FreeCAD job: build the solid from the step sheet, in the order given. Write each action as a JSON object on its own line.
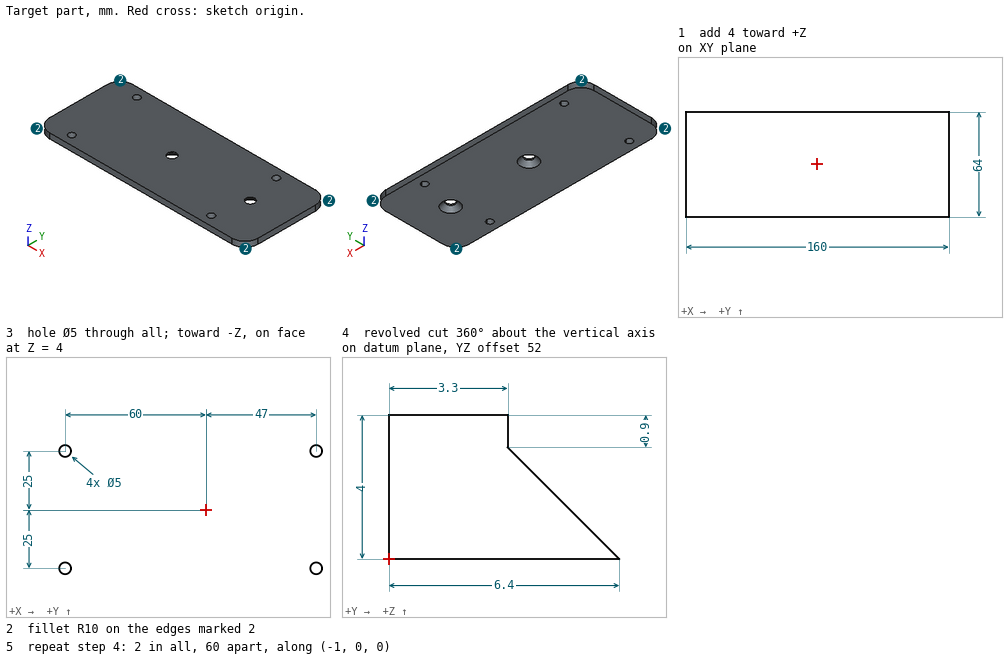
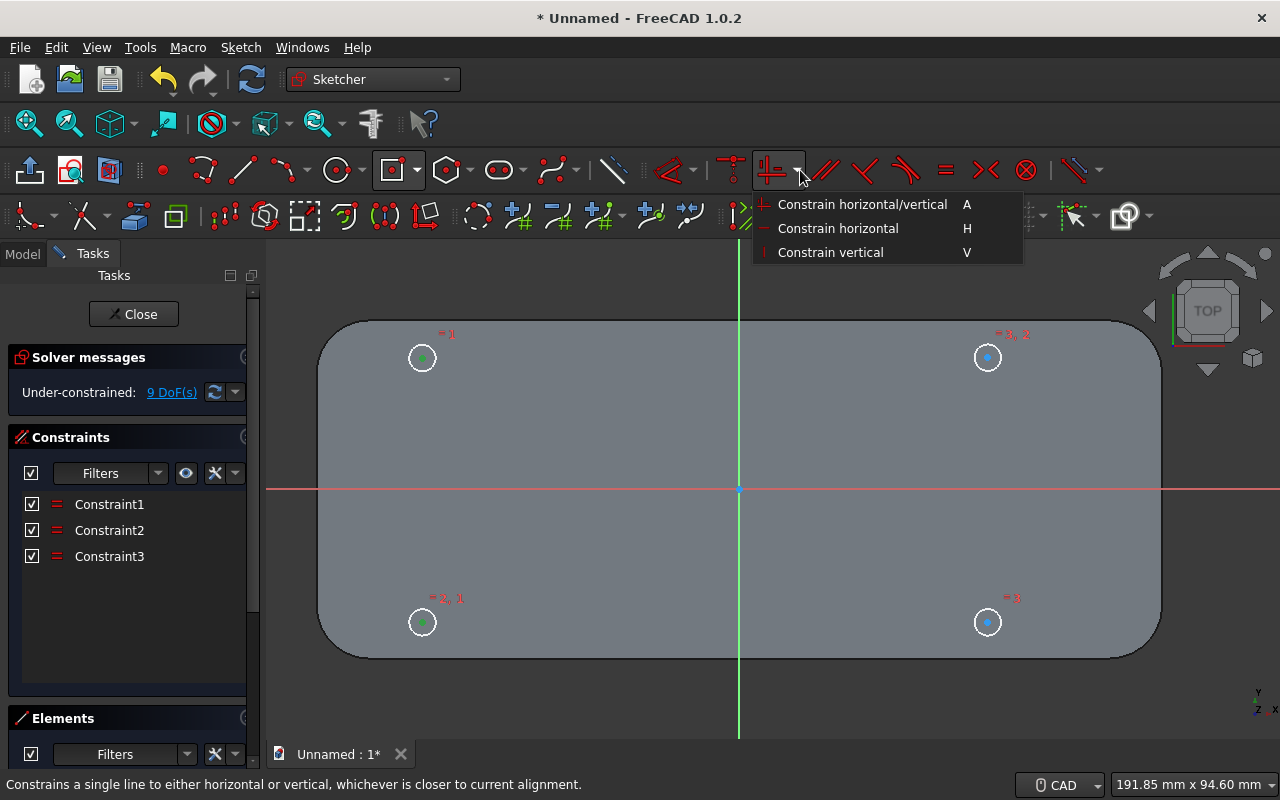
{"action": "left_click", "coordinate": [888, 252]}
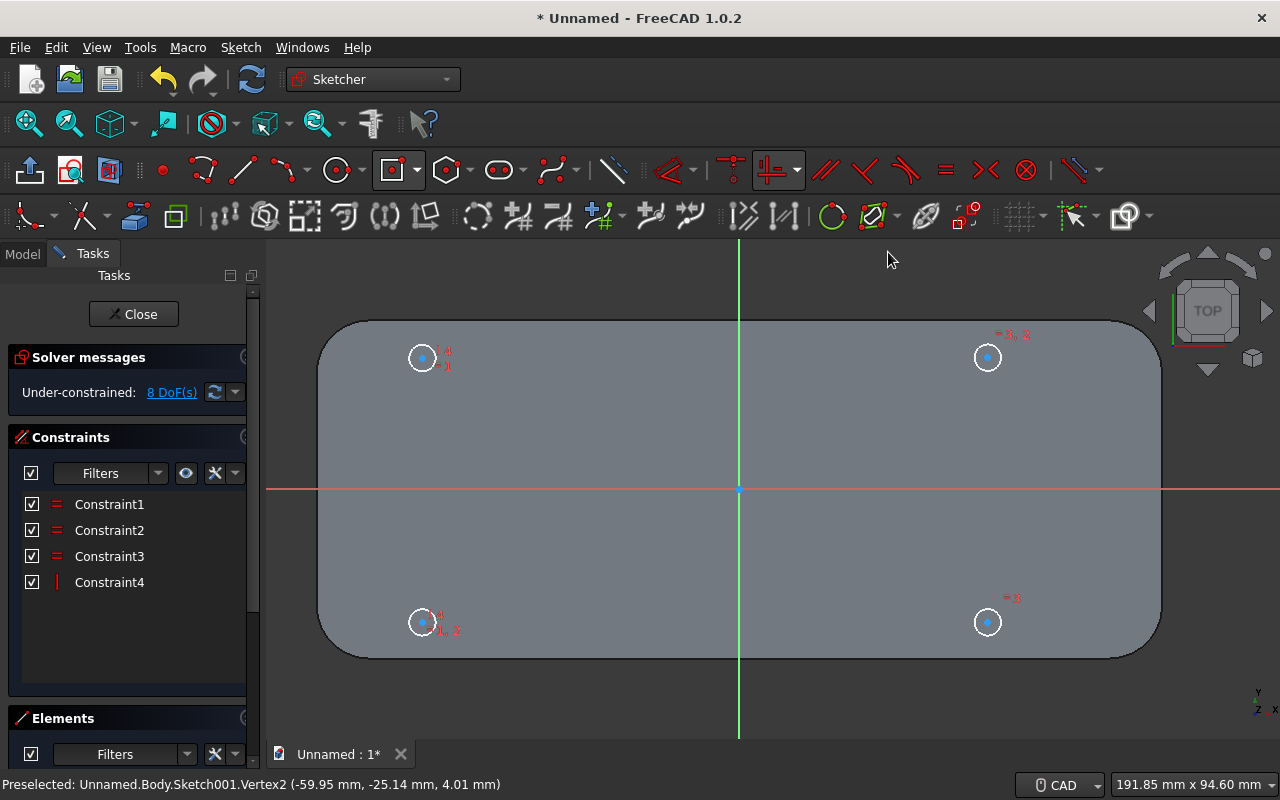
{"action": "left_click", "coordinate": [422, 358]}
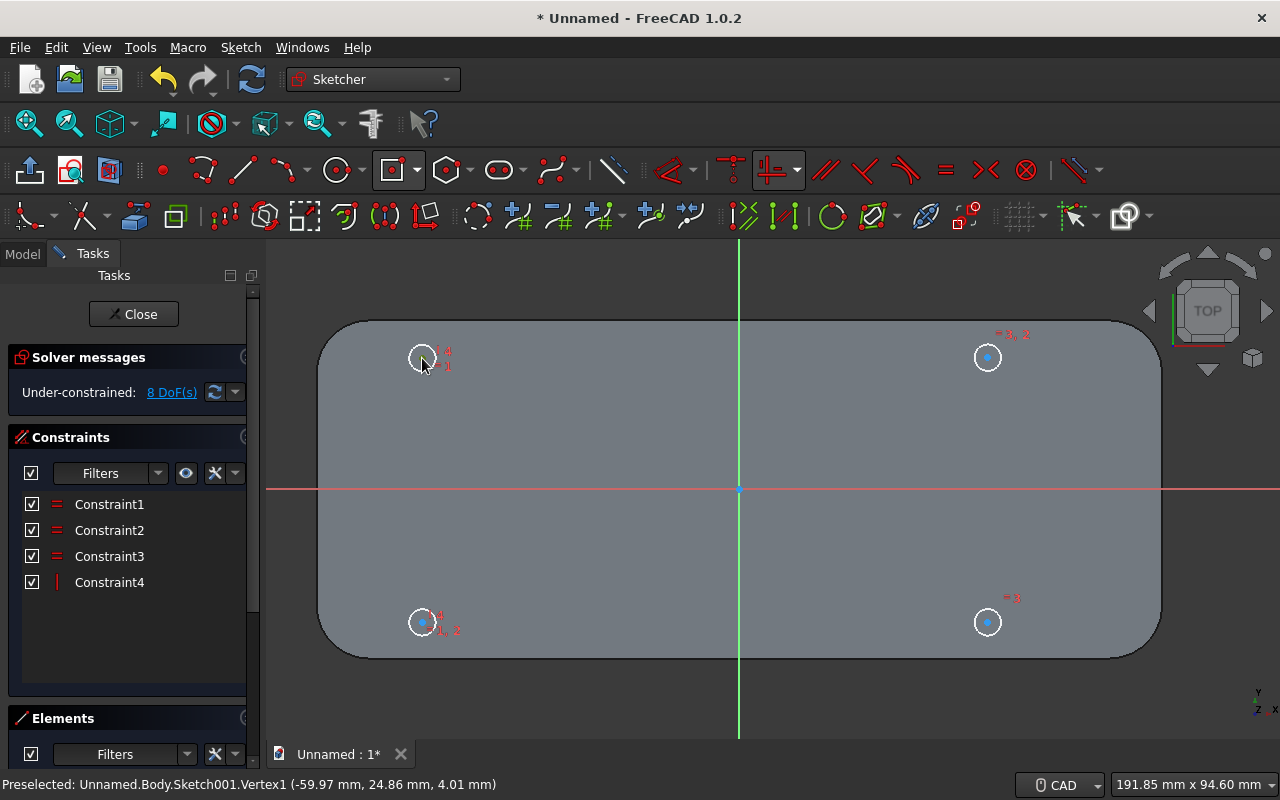
{"action": "left_click", "coordinate": [988, 358]}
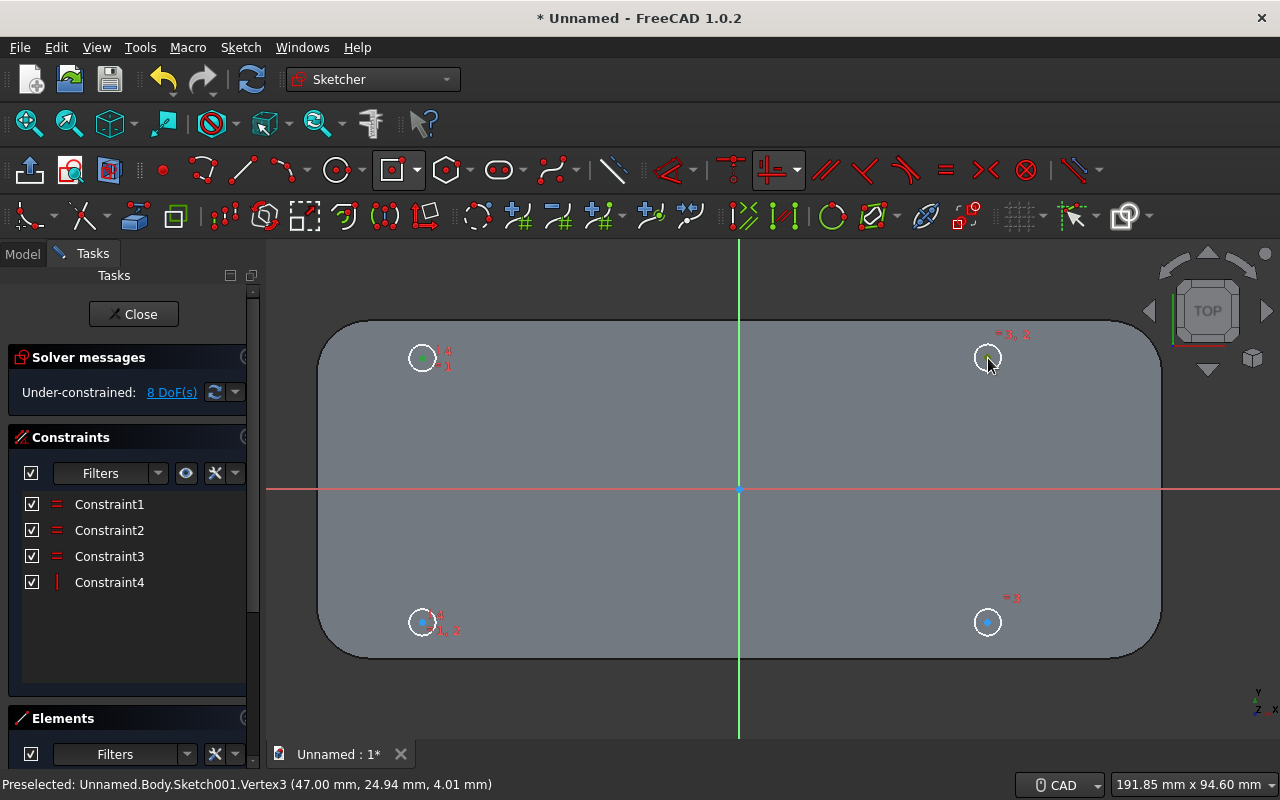
{"action": "key", "text": "h"}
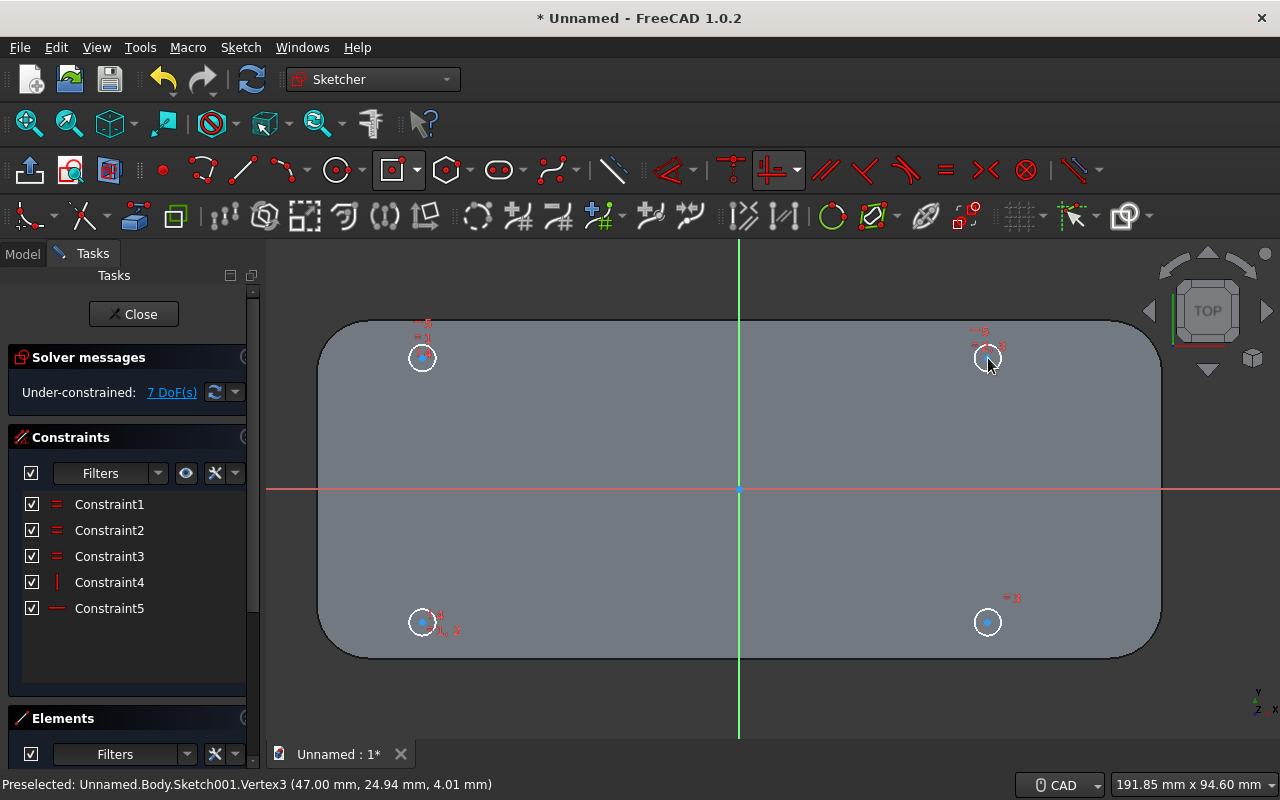
{"action": "left_click", "coordinate": [988, 358]}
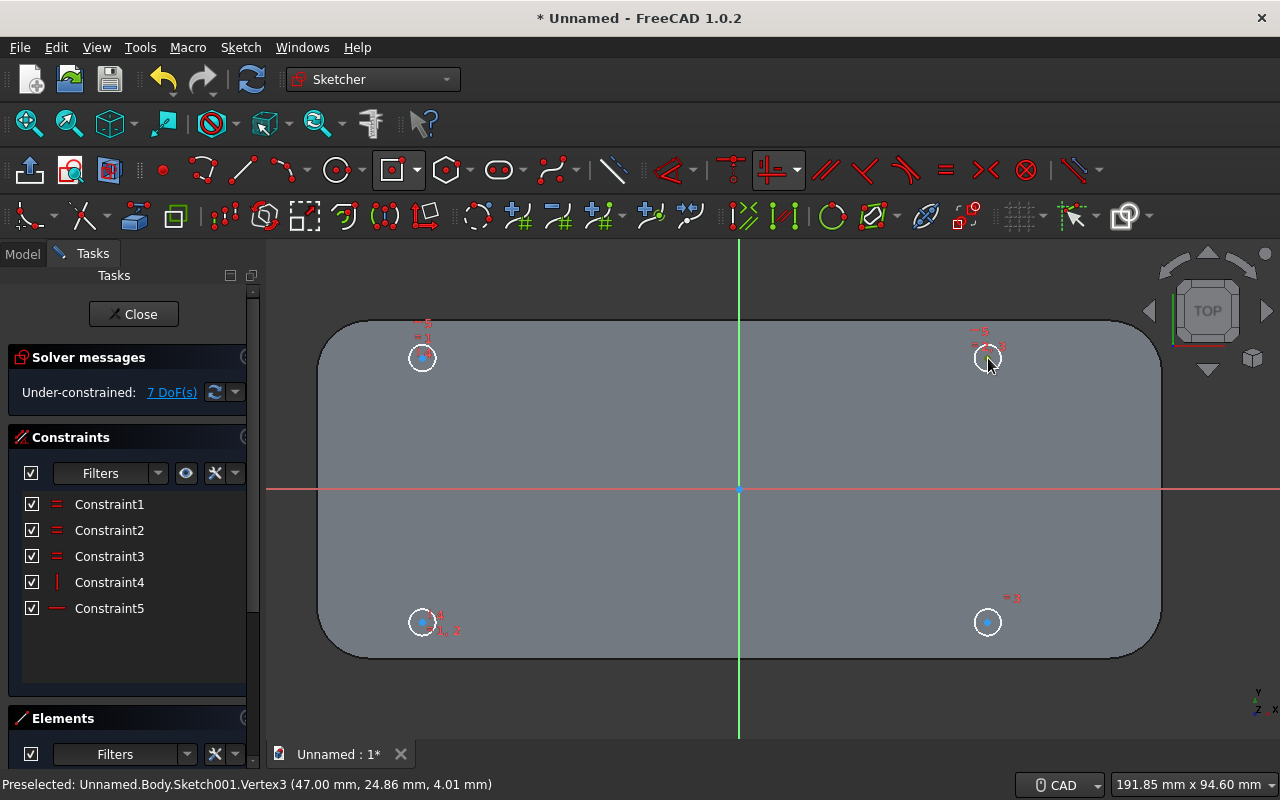
{"action": "left_click", "coordinate": [988, 622]}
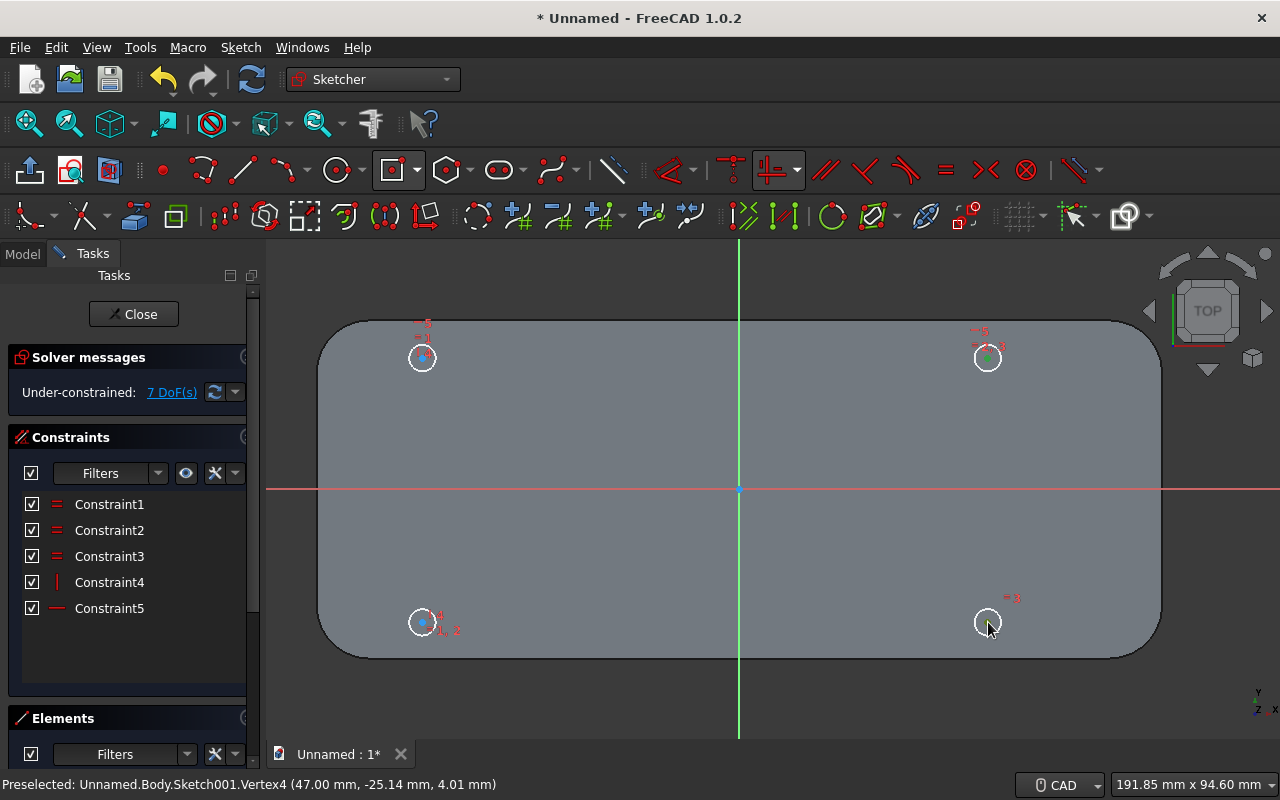
{"action": "key", "text": "v"}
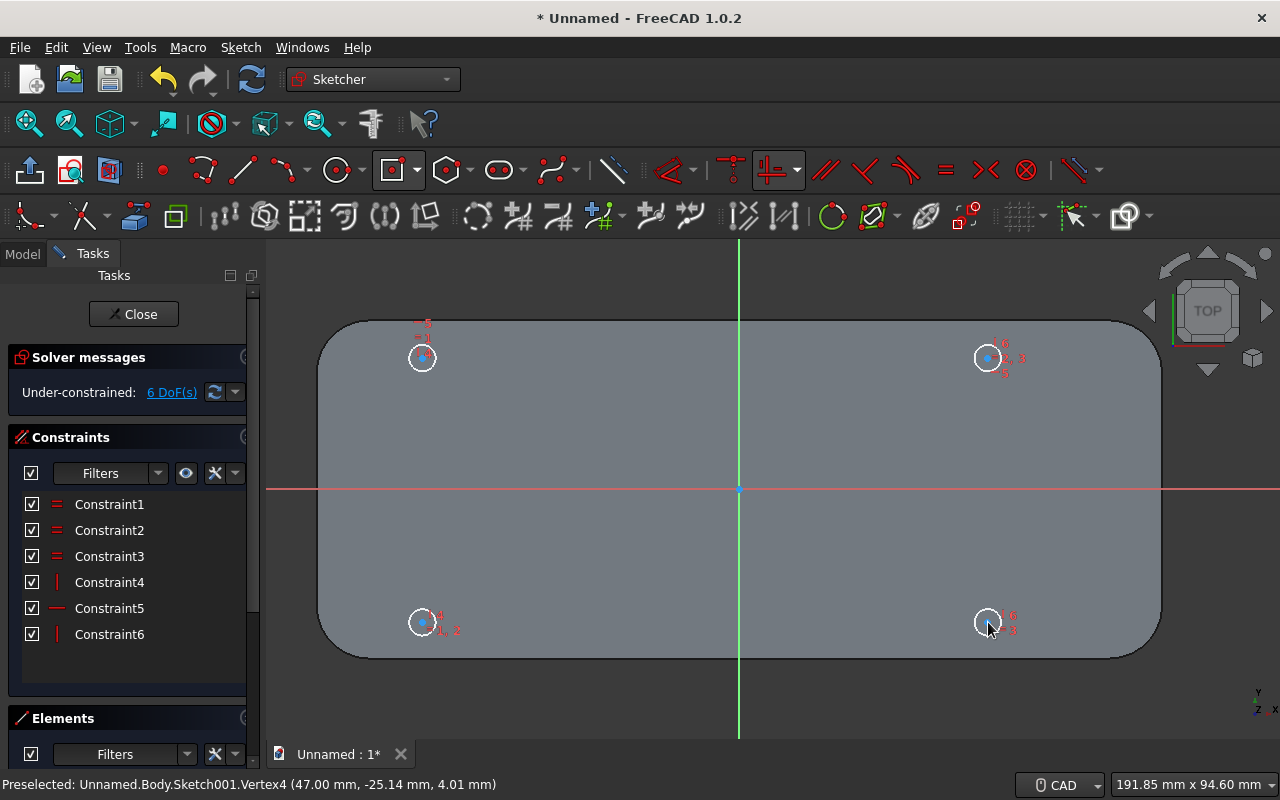
{"action": "left_click", "coordinate": [422, 622]}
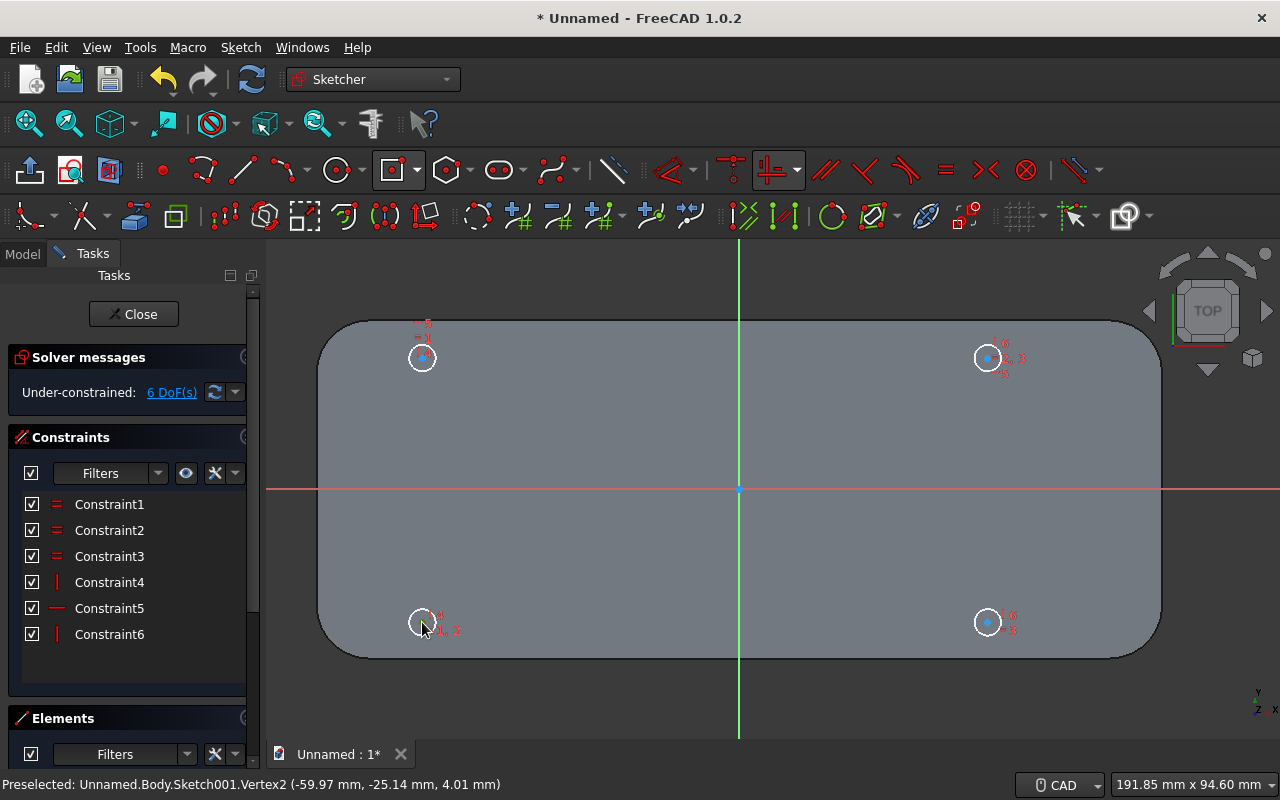
{"action": "left_click", "coordinate": [988, 622]}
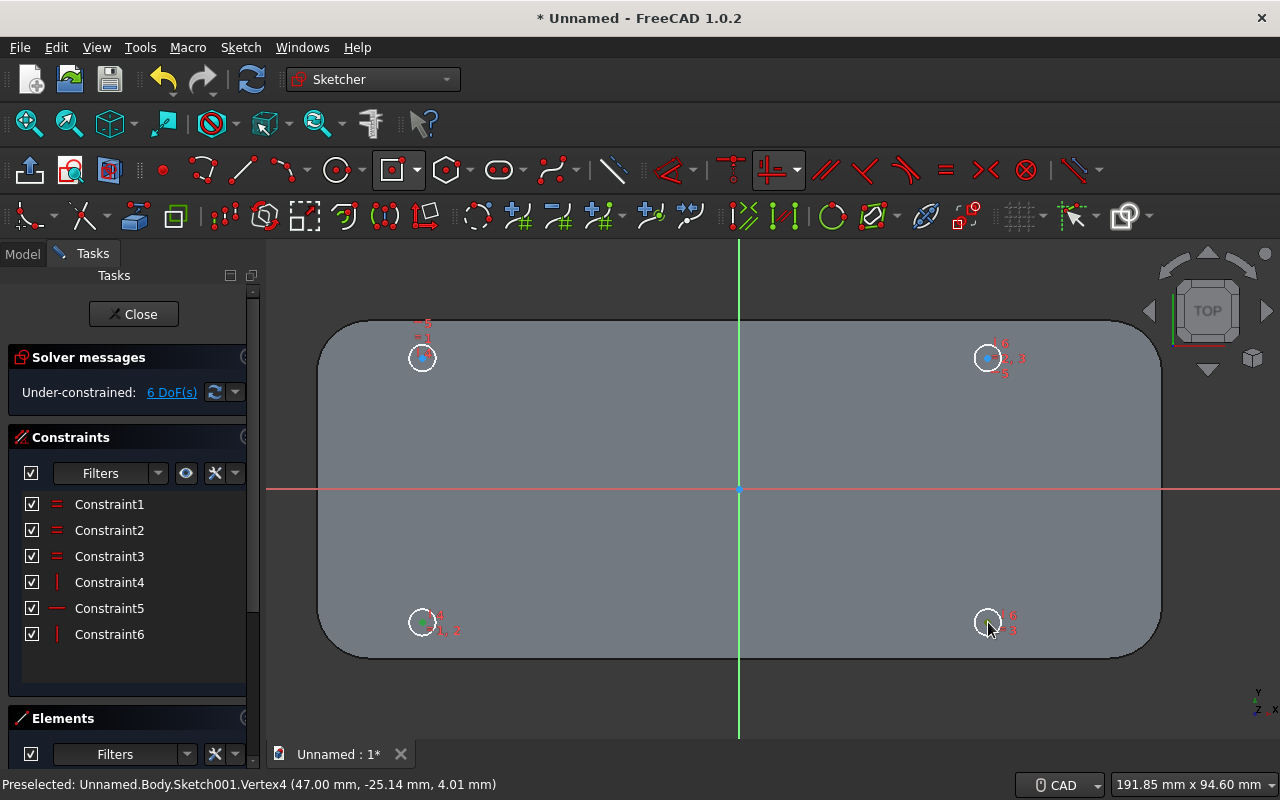
{"action": "left_click", "coordinate": [800, 170]}